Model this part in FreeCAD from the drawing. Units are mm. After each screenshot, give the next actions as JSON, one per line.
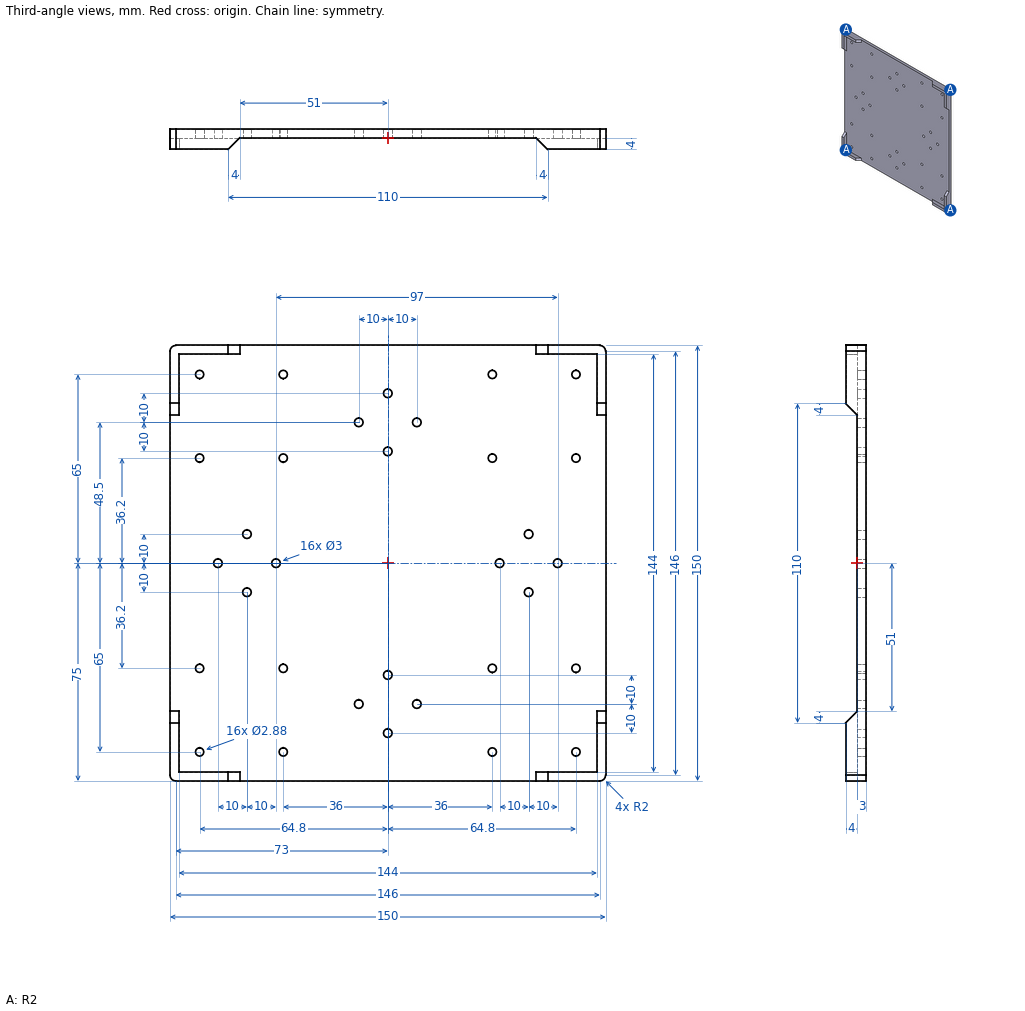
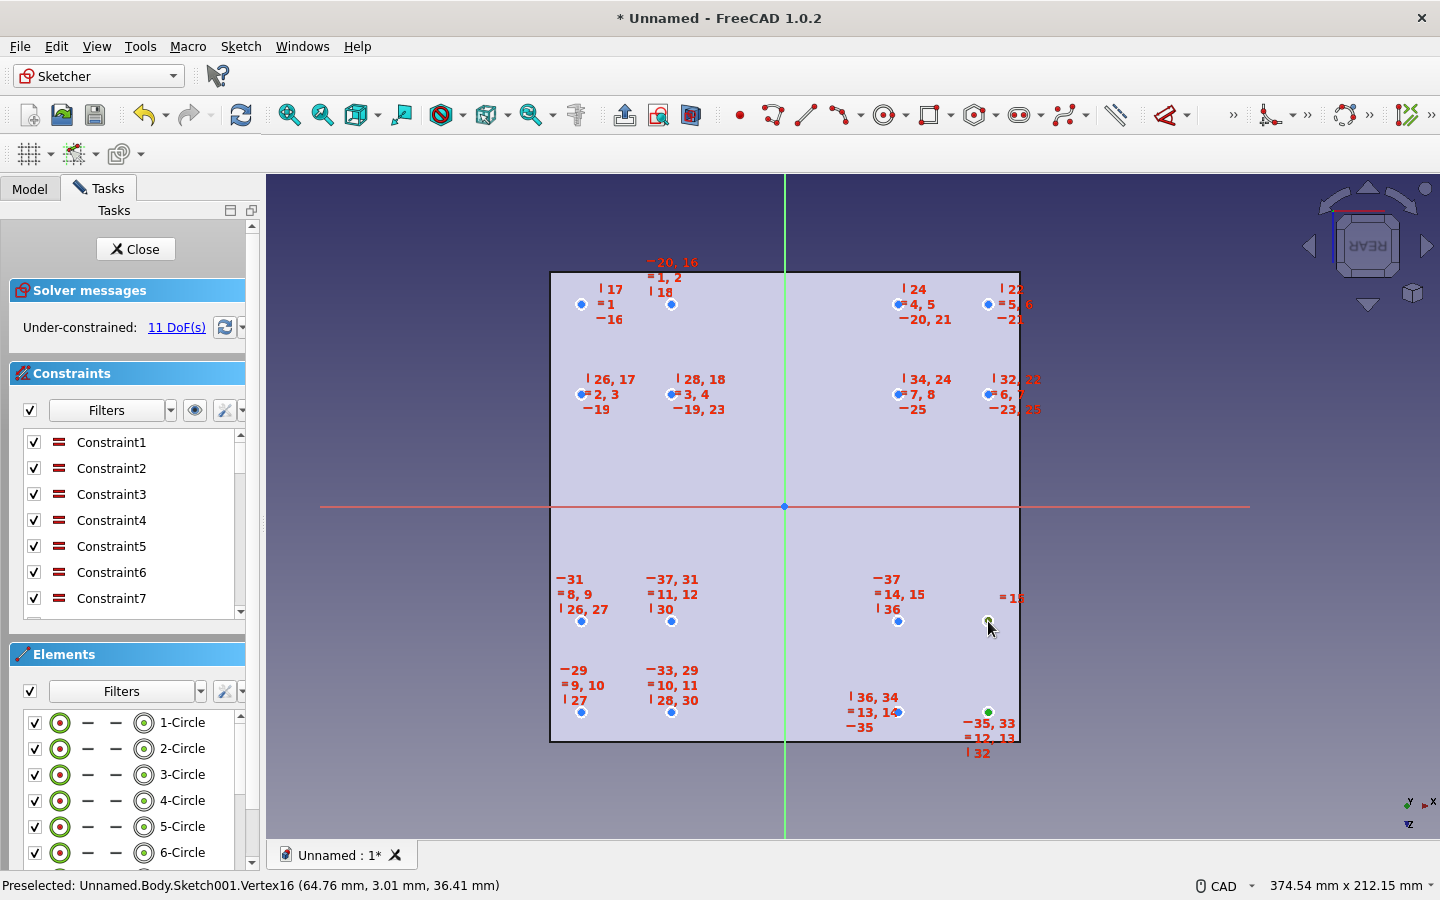
{"action": "key", "text": "v"}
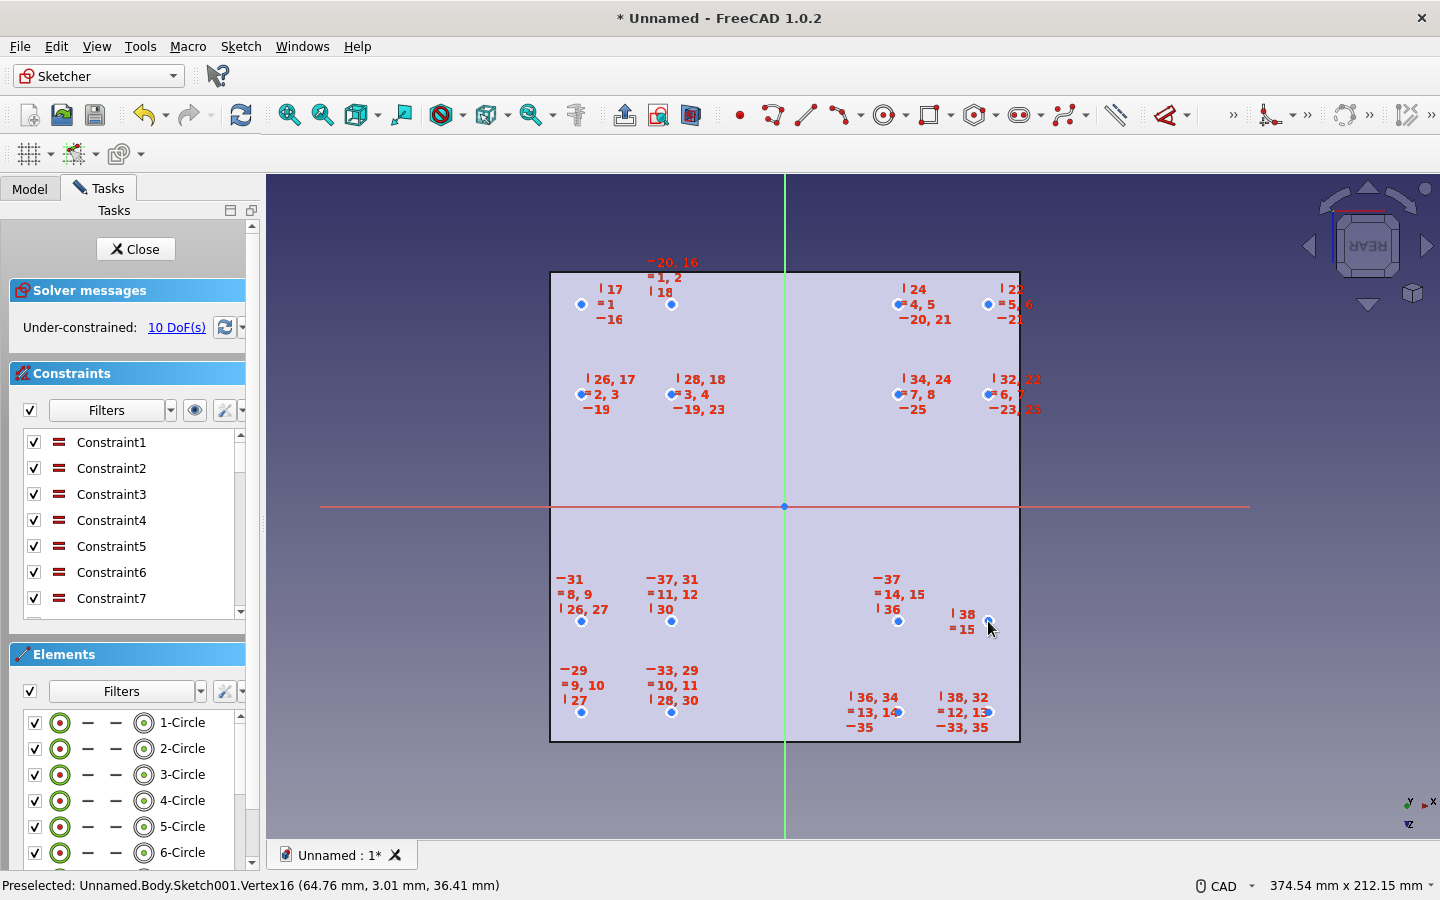
{"action": "left_click", "coordinate": [898, 621]}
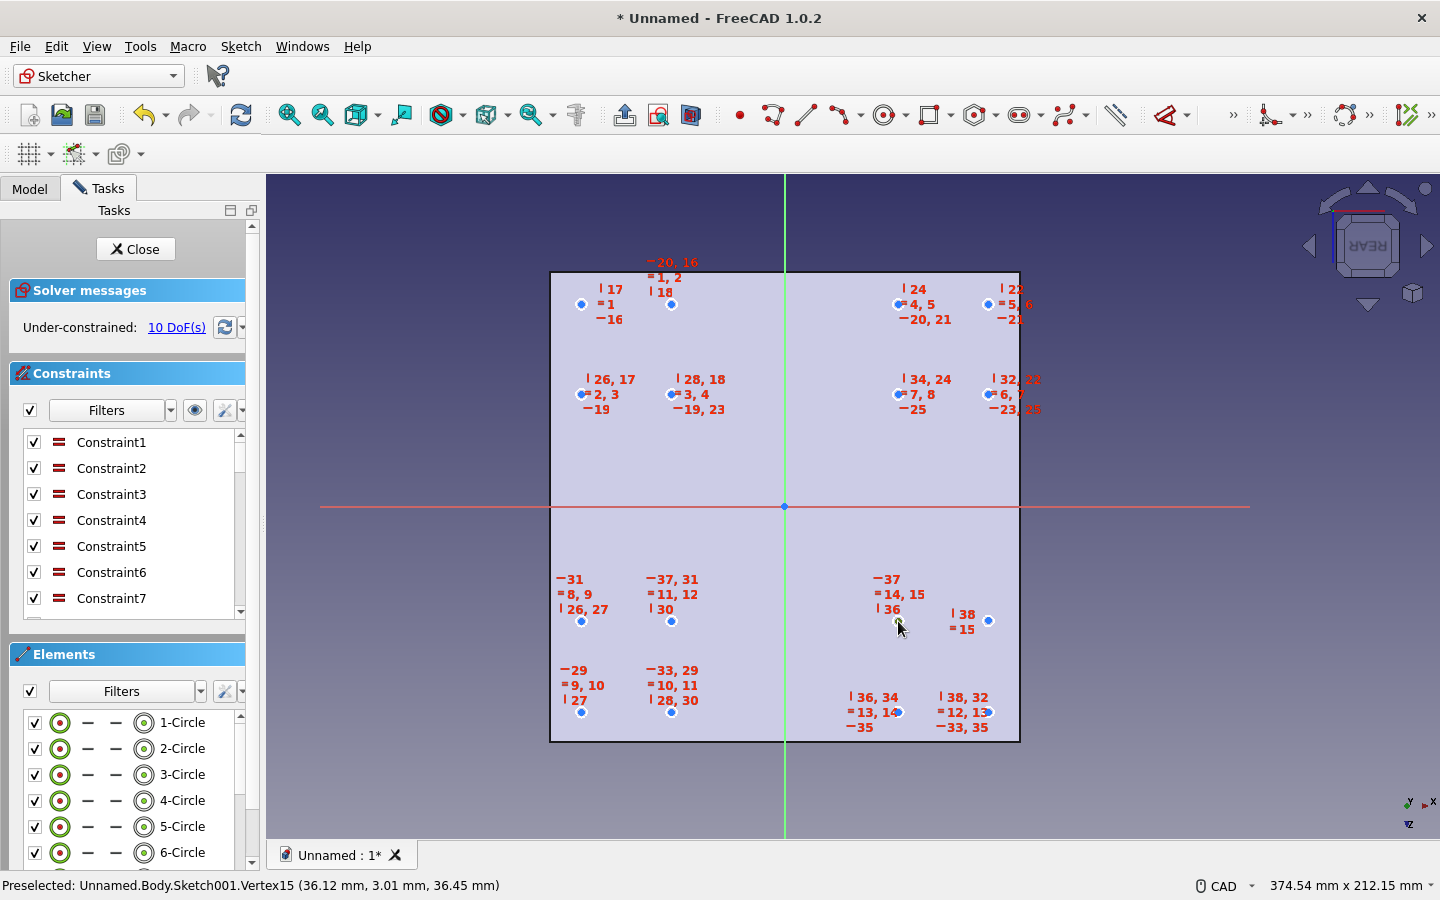
{"action": "left_click", "coordinate": [988, 621]}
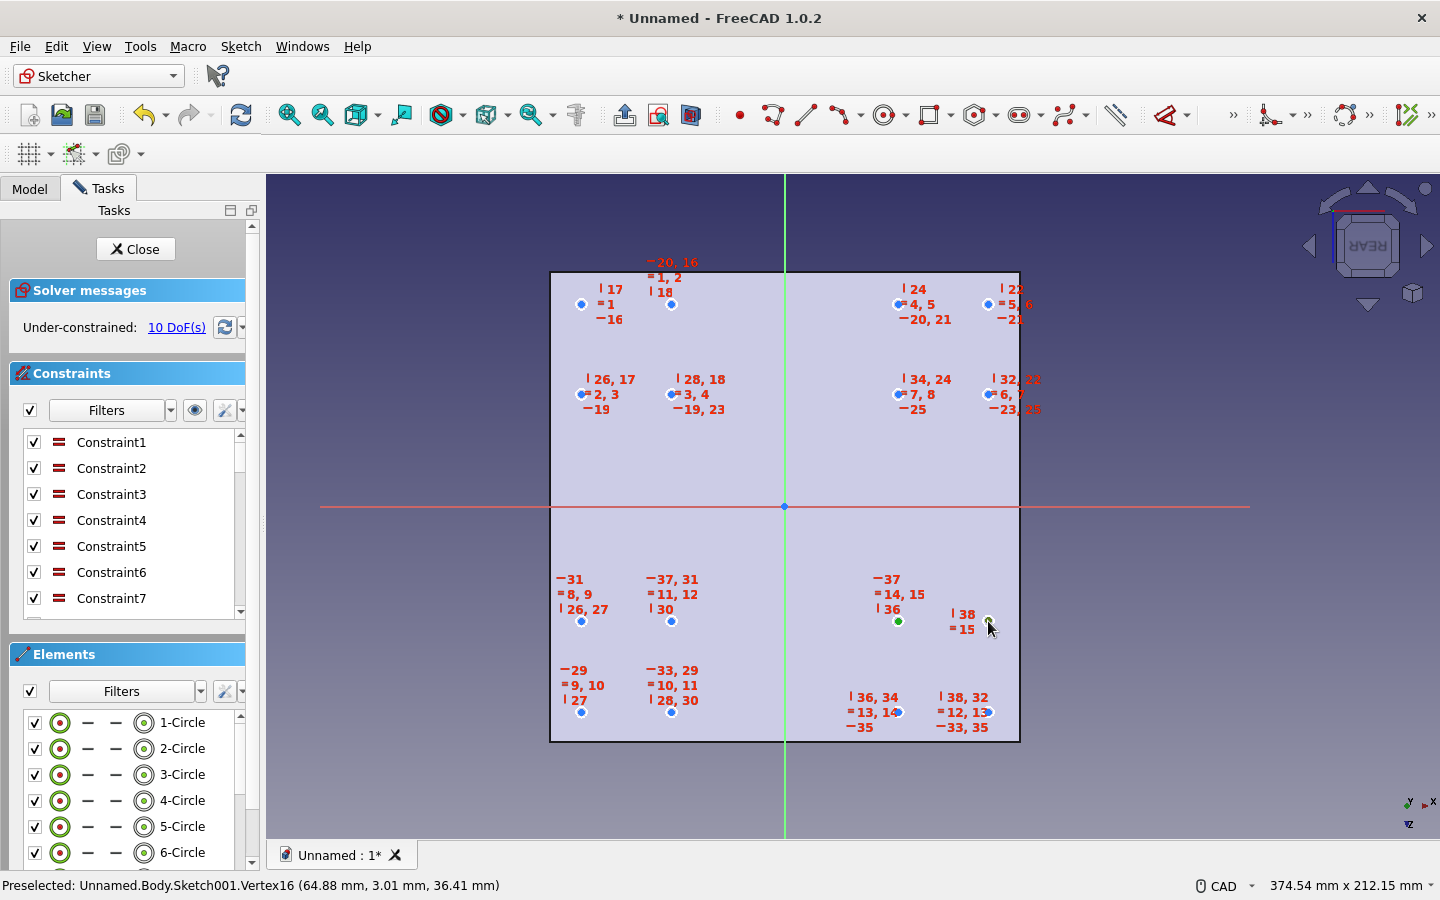
{"action": "key", "text": "h"}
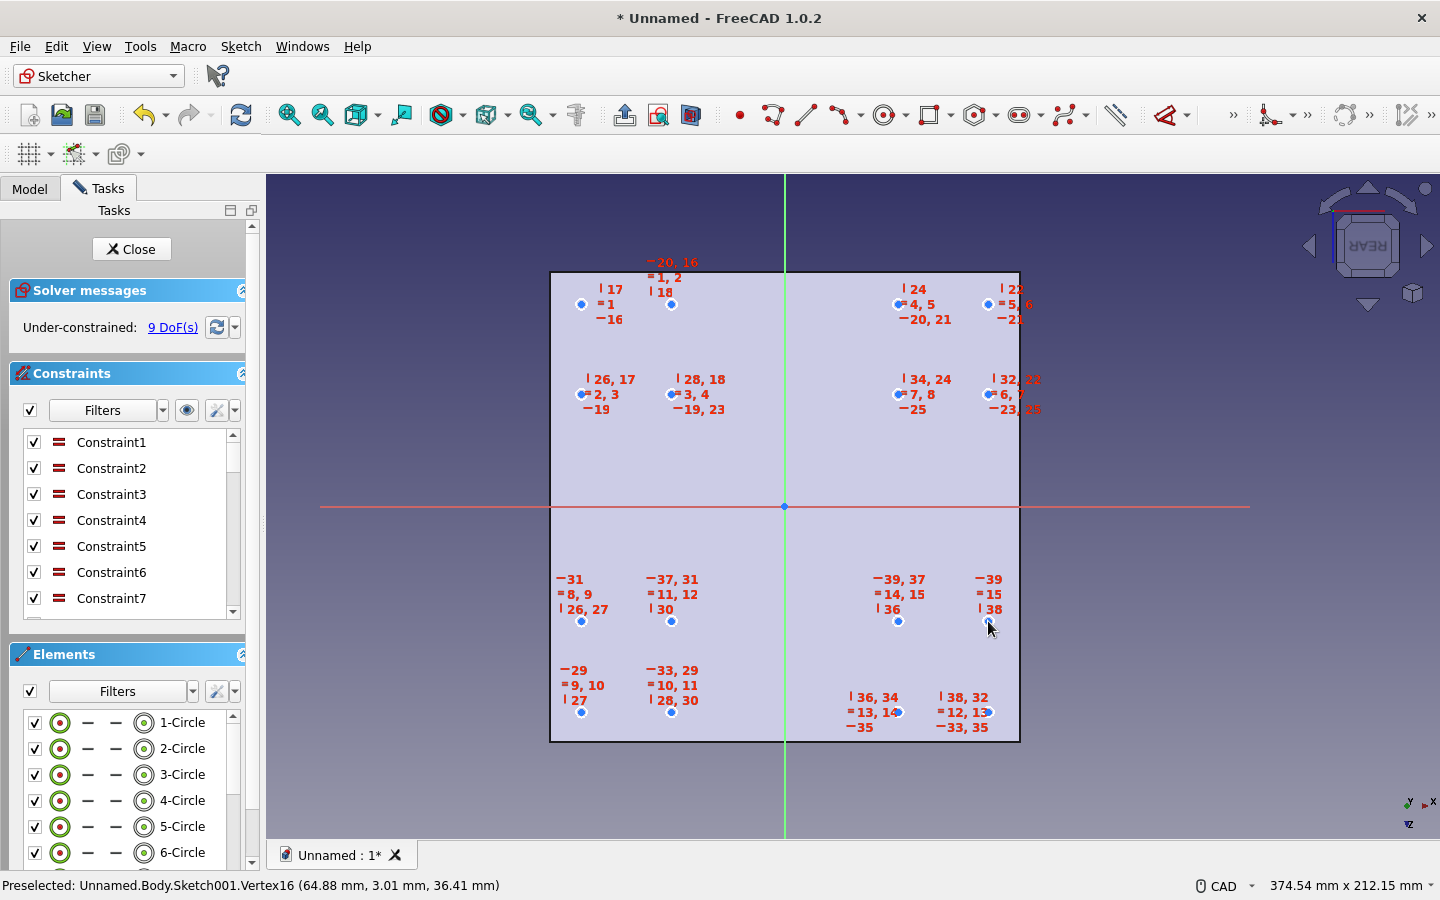
{"action": "left_click", "coordinate": [1164, 116]}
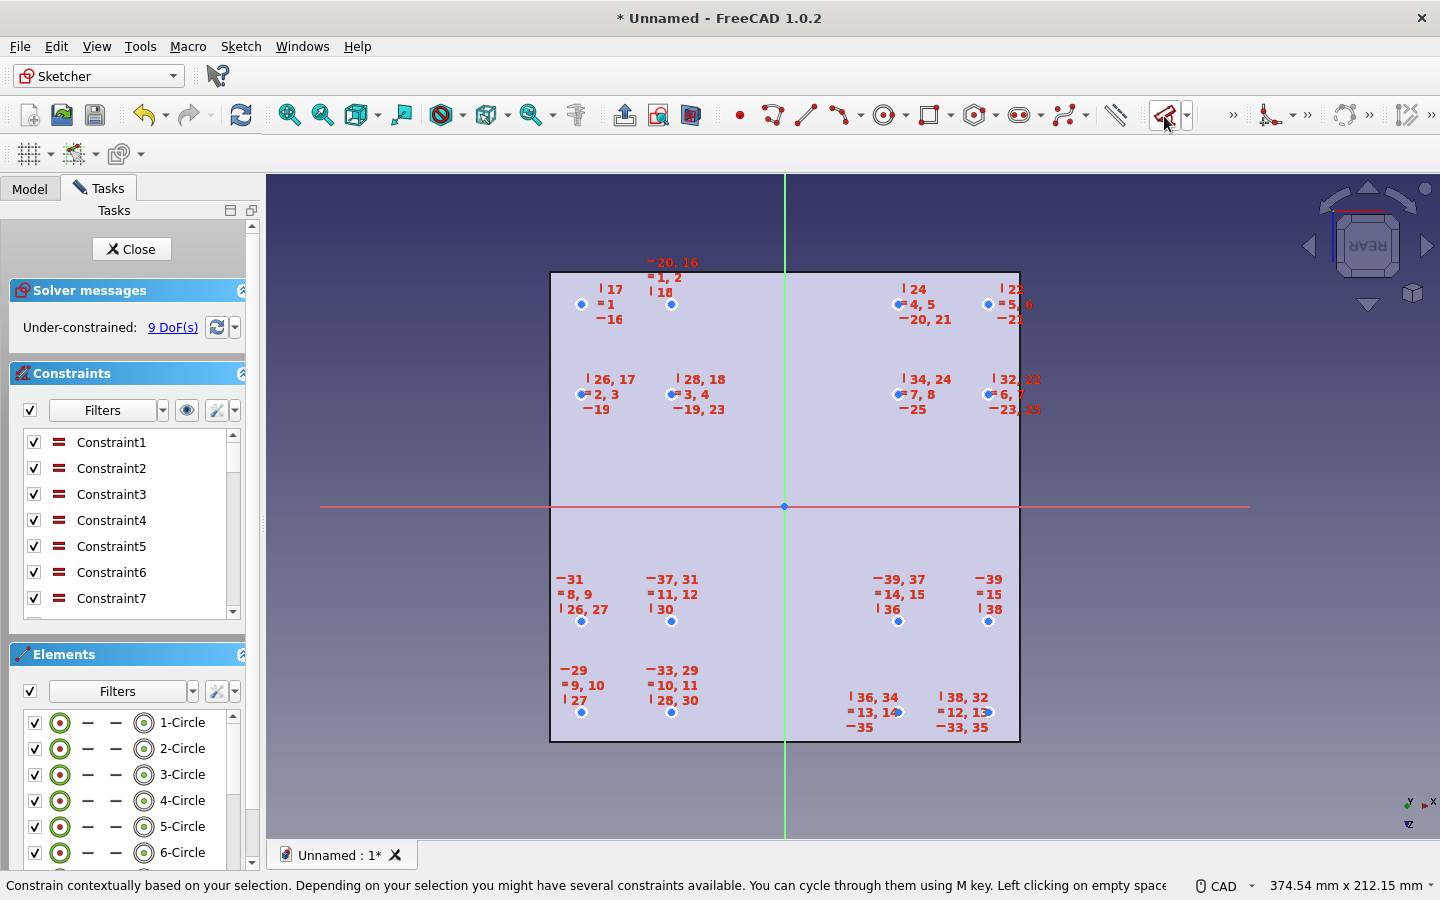
{"action": "scroll", "coordinate": [585, 301], "scroll_direction": "up", "scroll_amount": 8}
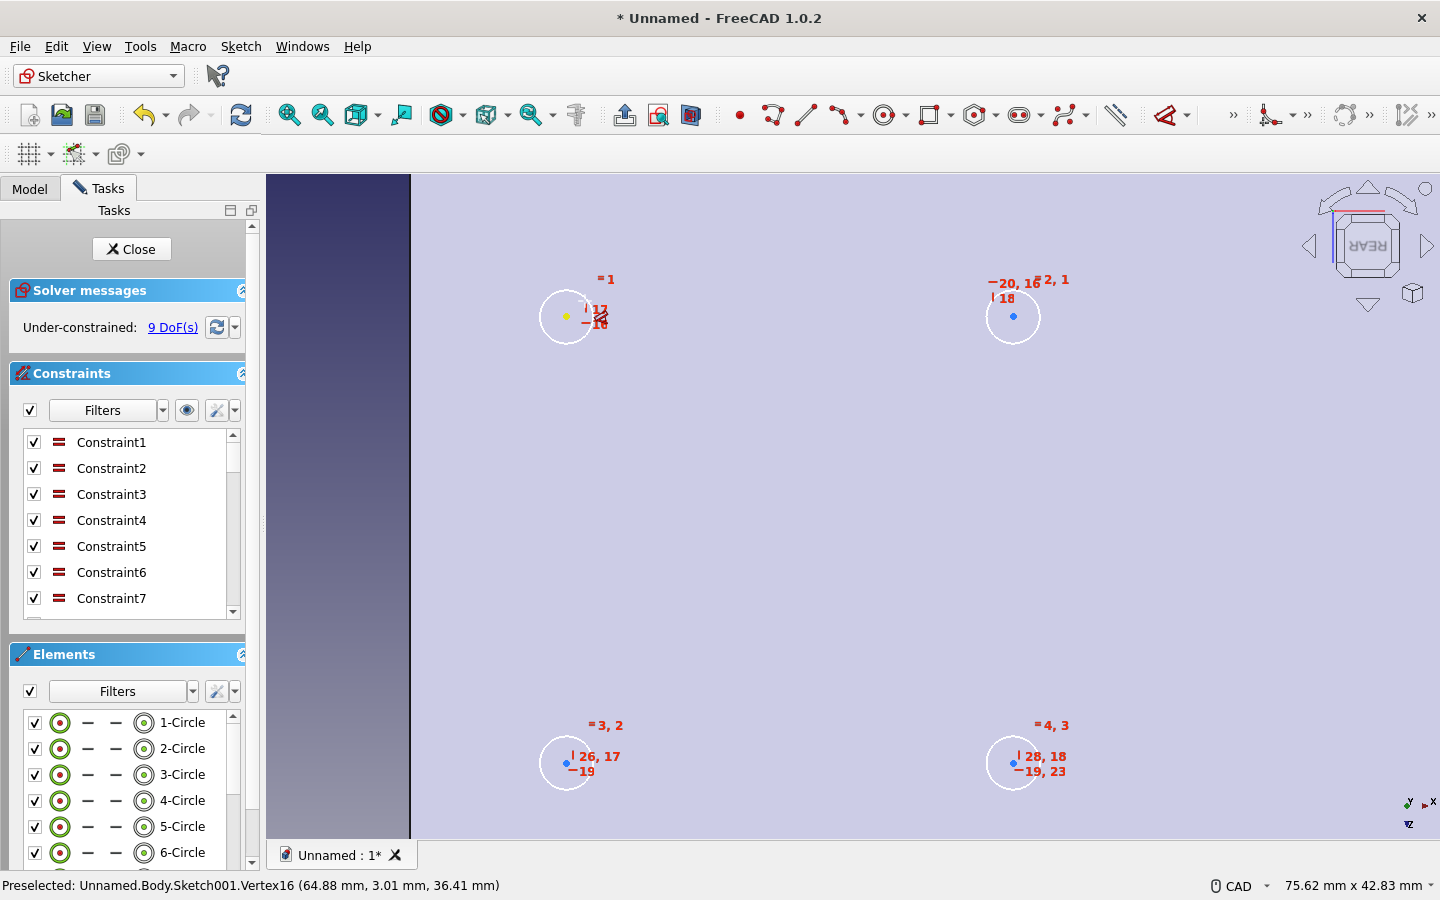
{"action": "left_click", "coordinate": [585, 298]}
{"action": "left_click", "coordinate": [607, 275]}